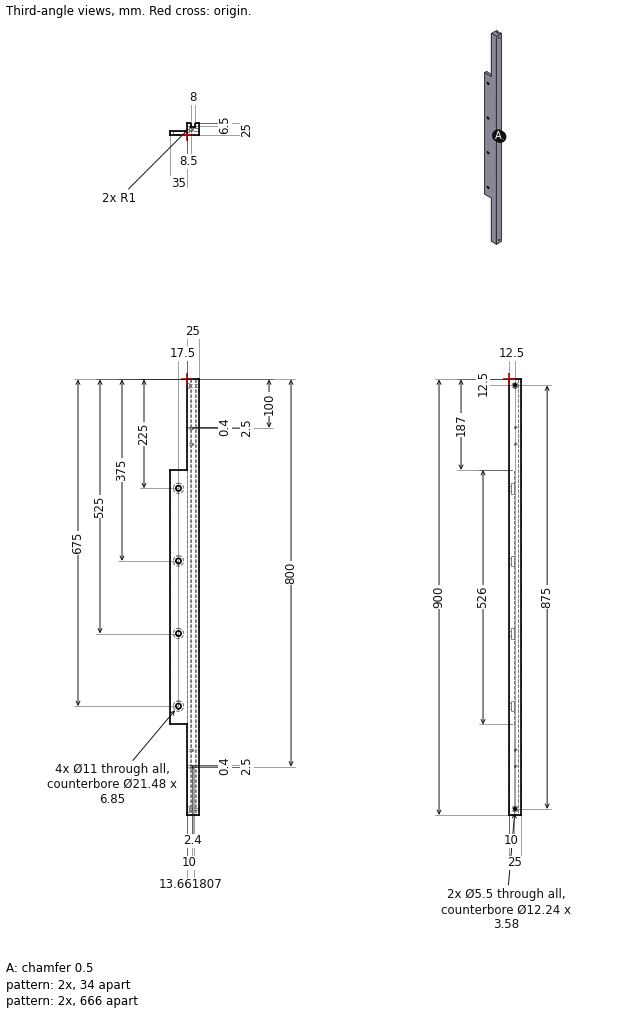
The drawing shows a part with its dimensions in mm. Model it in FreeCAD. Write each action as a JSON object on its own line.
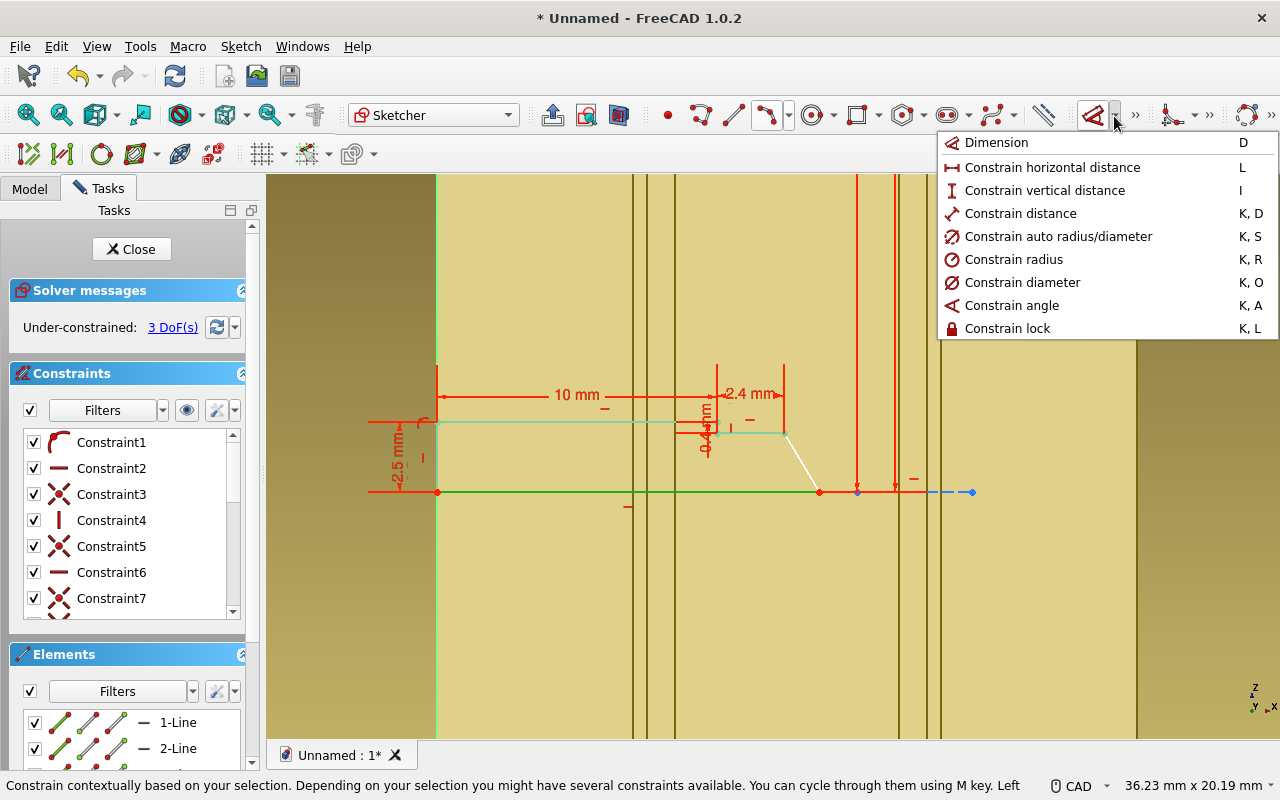
{"action": "left_click", "coordinate": [1108, 168]}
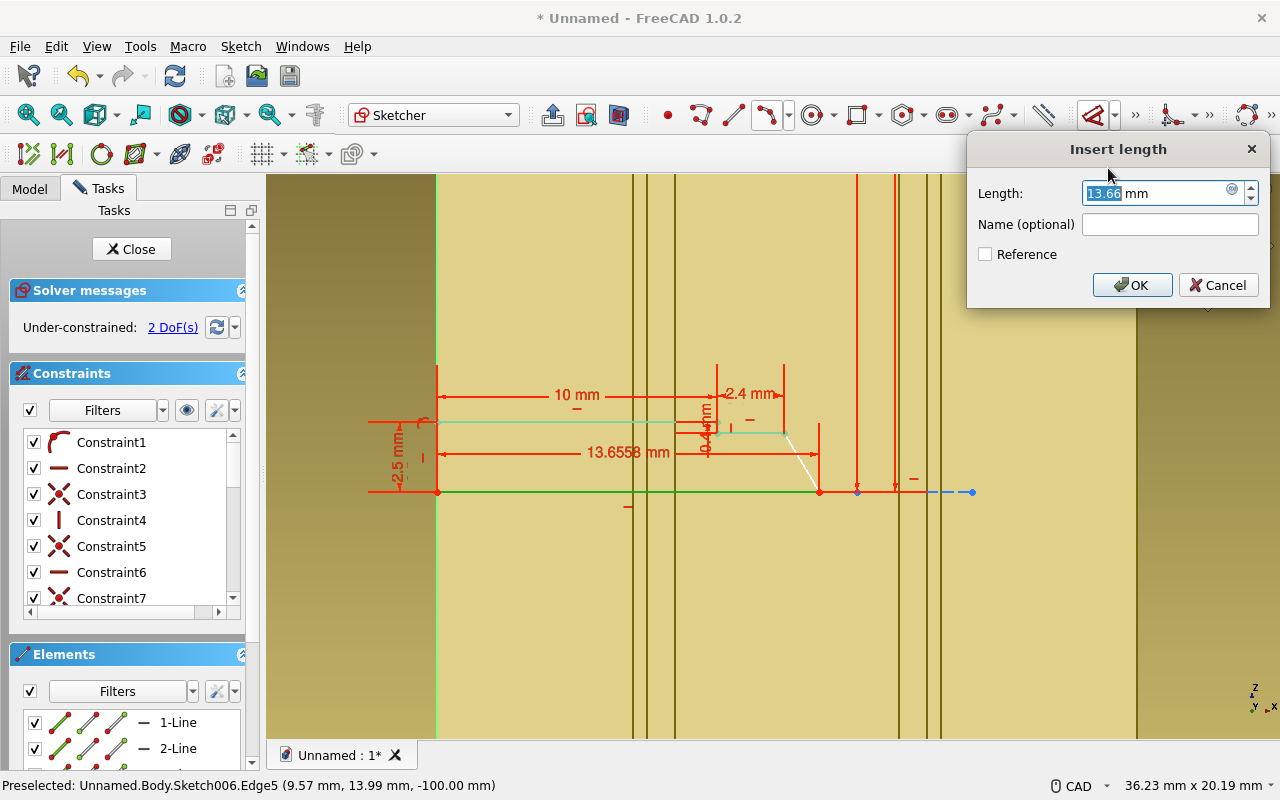
{"action": "type", "text": "13.661807"}
{"action": "key", "text": "Return"}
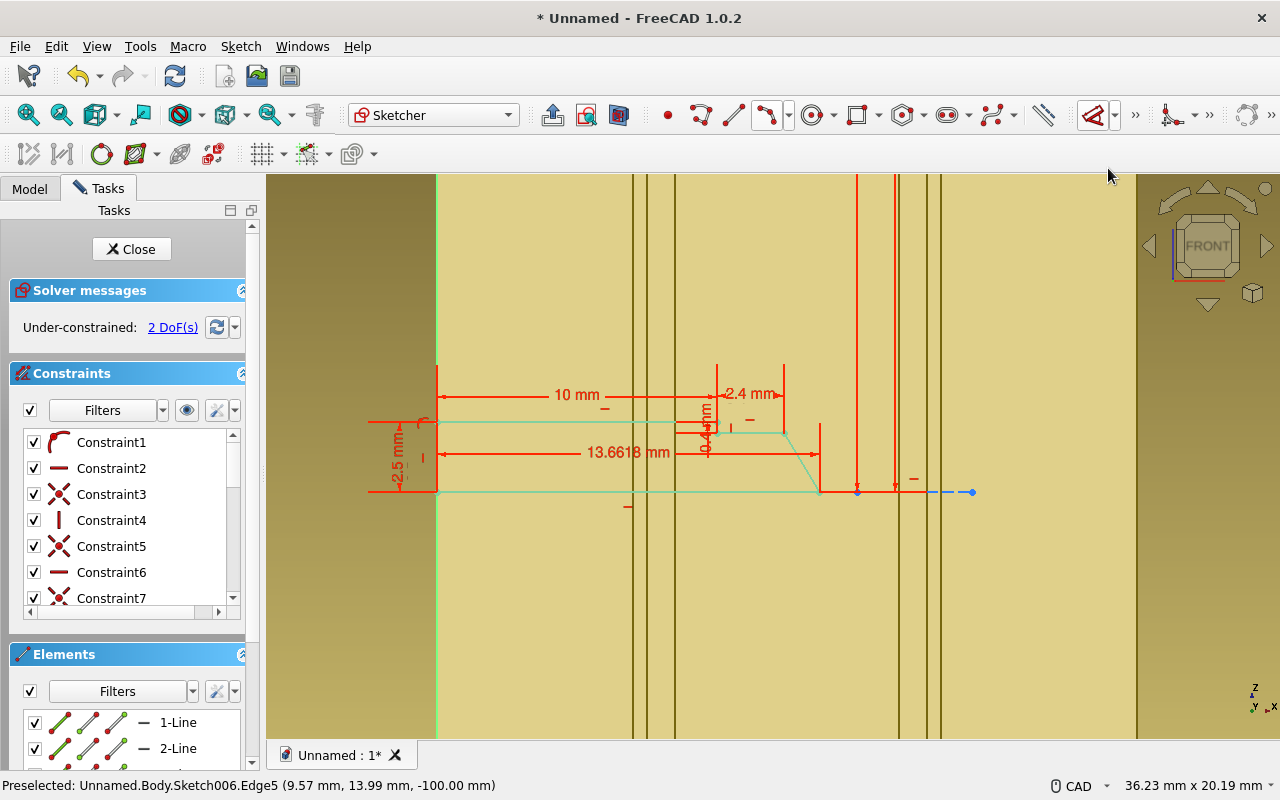
{"action": "left_click", "coordinate": [132, 249]}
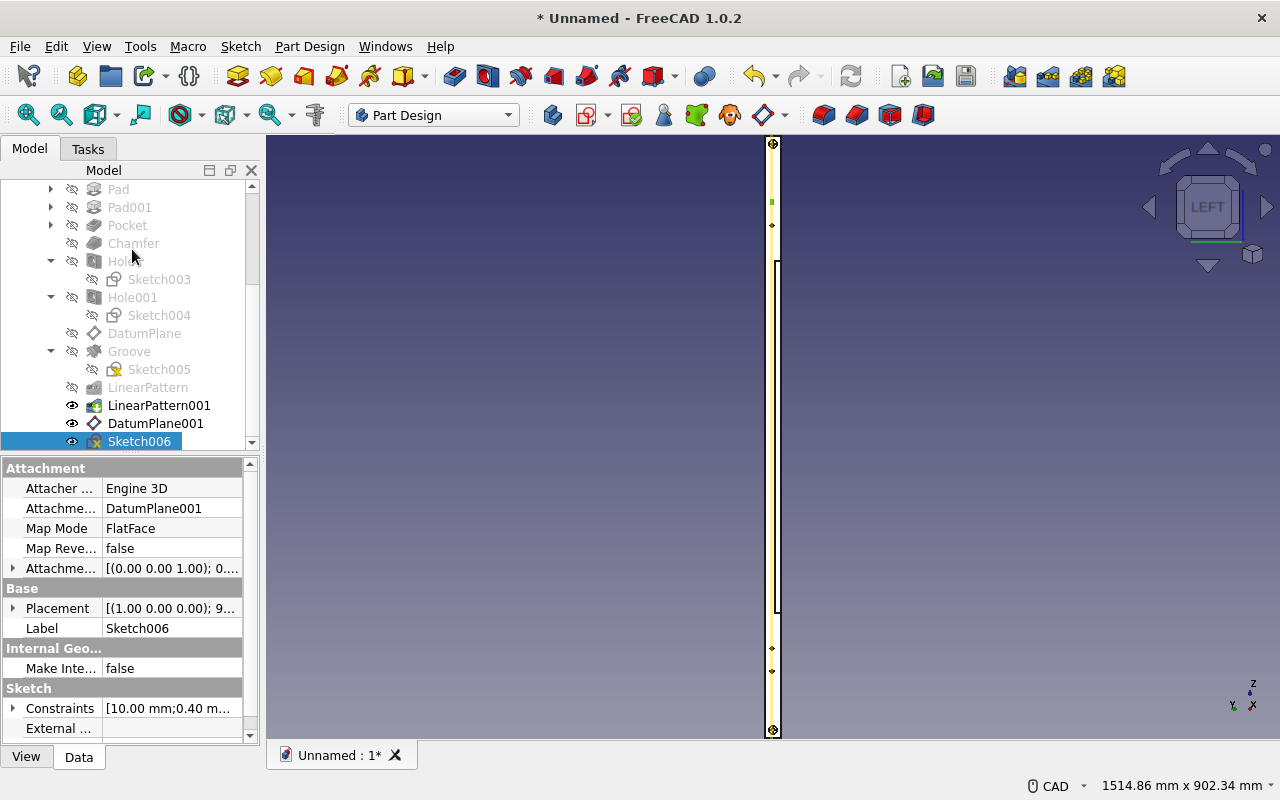
{"action": "left_click", "coordinate": [521, 76]}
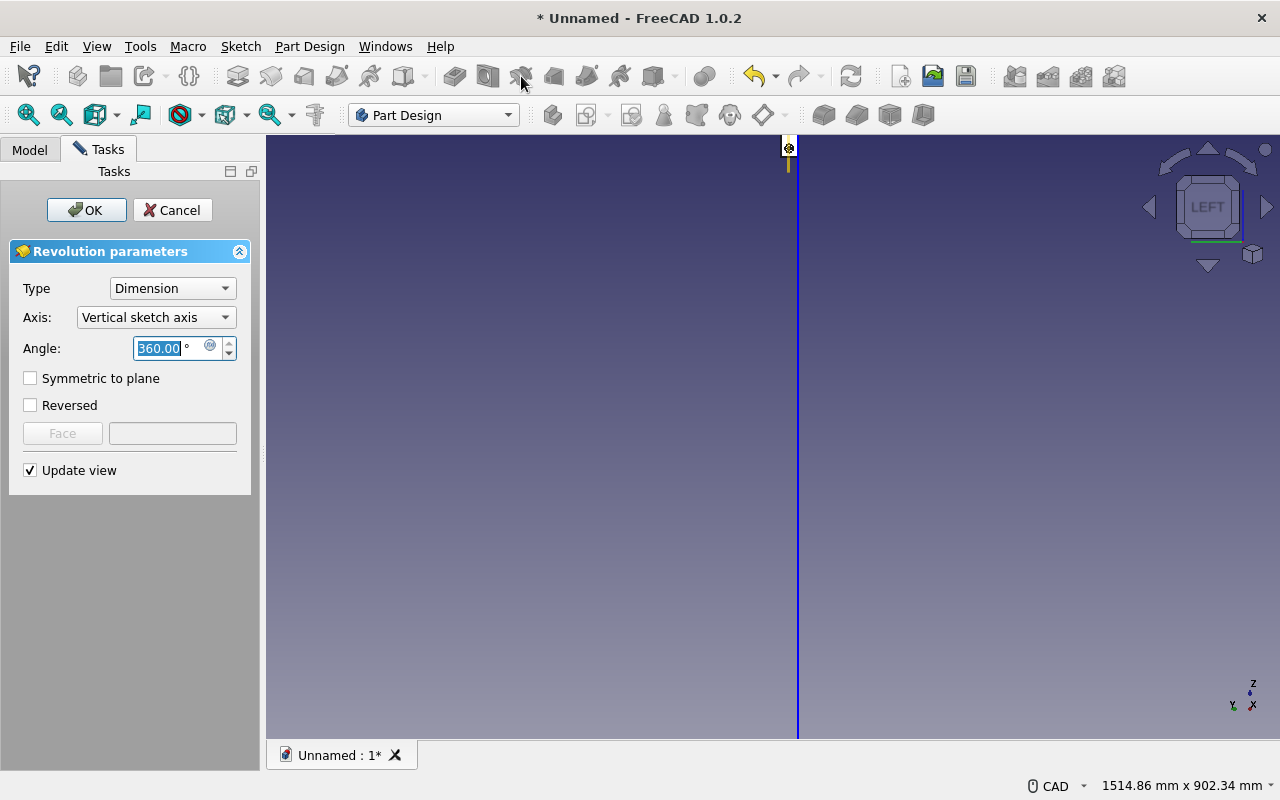
{"action": "left_click", "coordinate": [157, 318]}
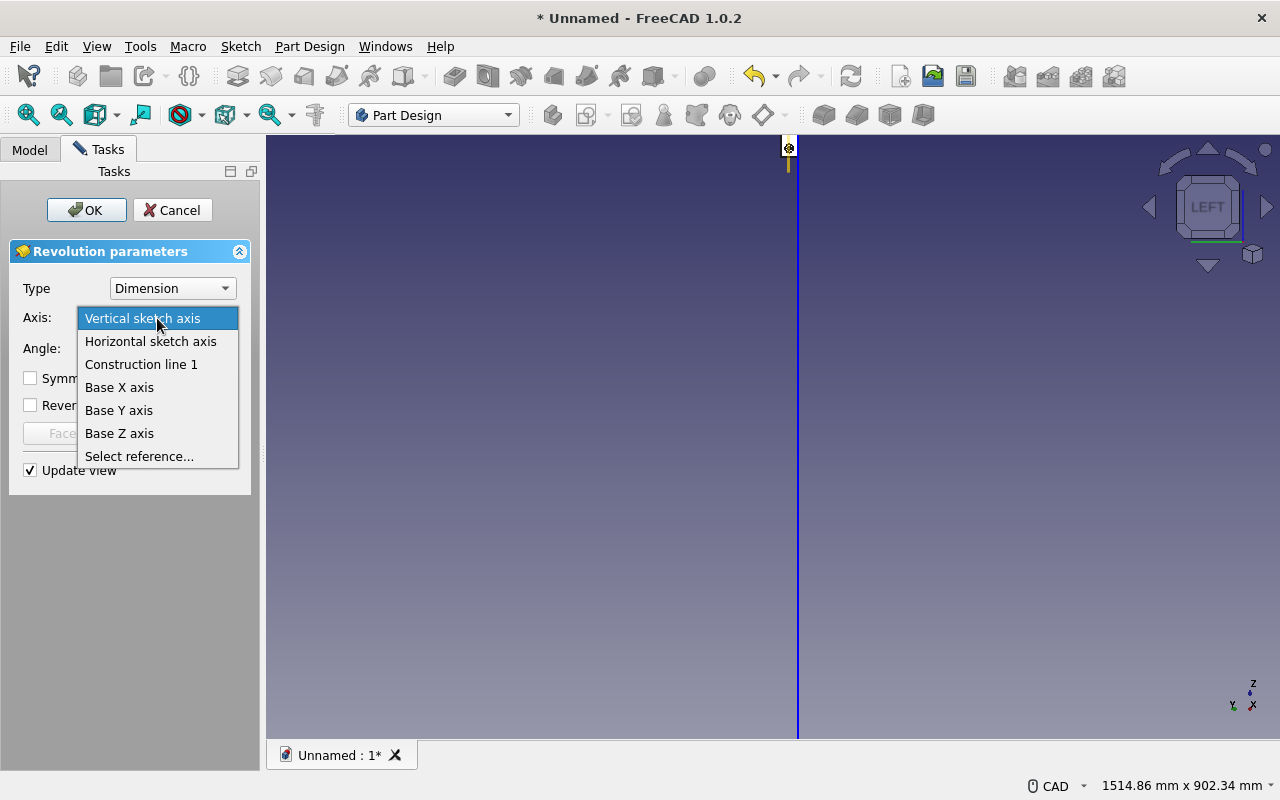
{"action": "left_click", "coordinate": [156, 364]}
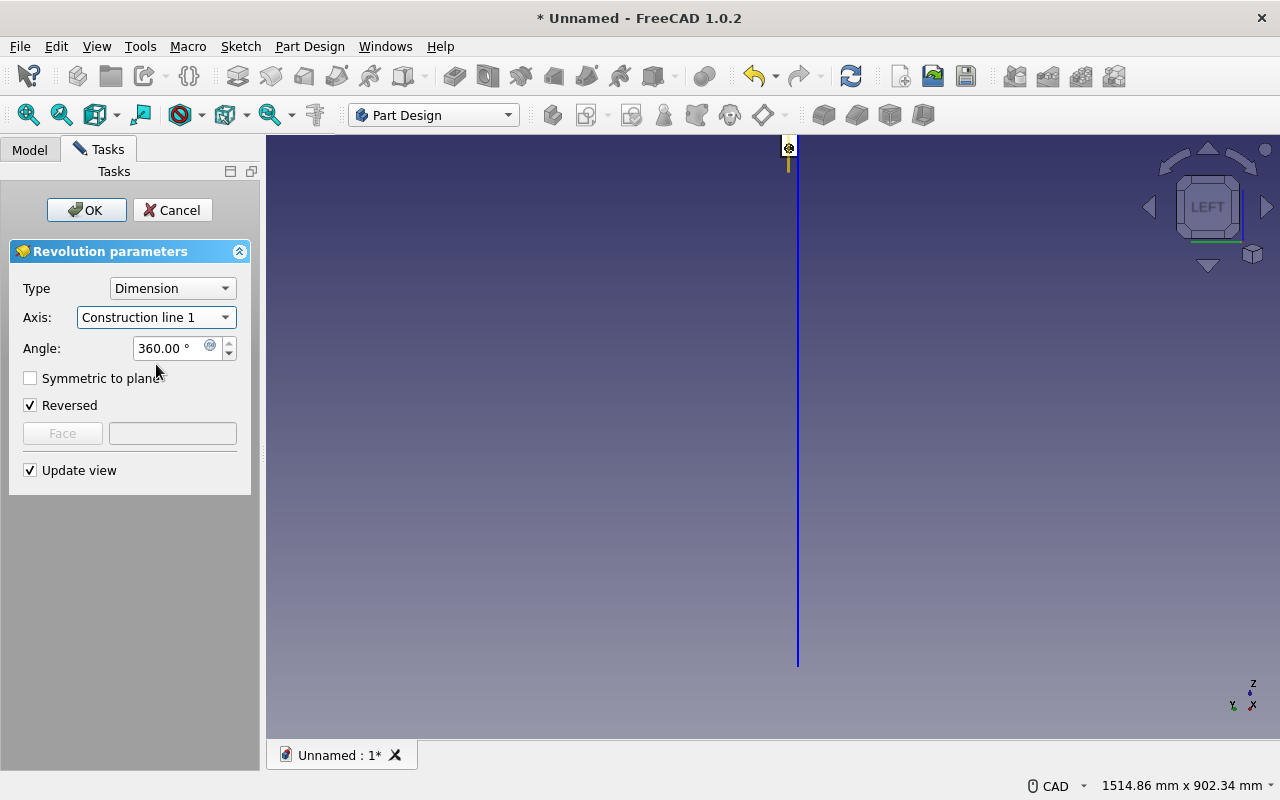
{"action": "left_click", "coordinate": [87, 210]}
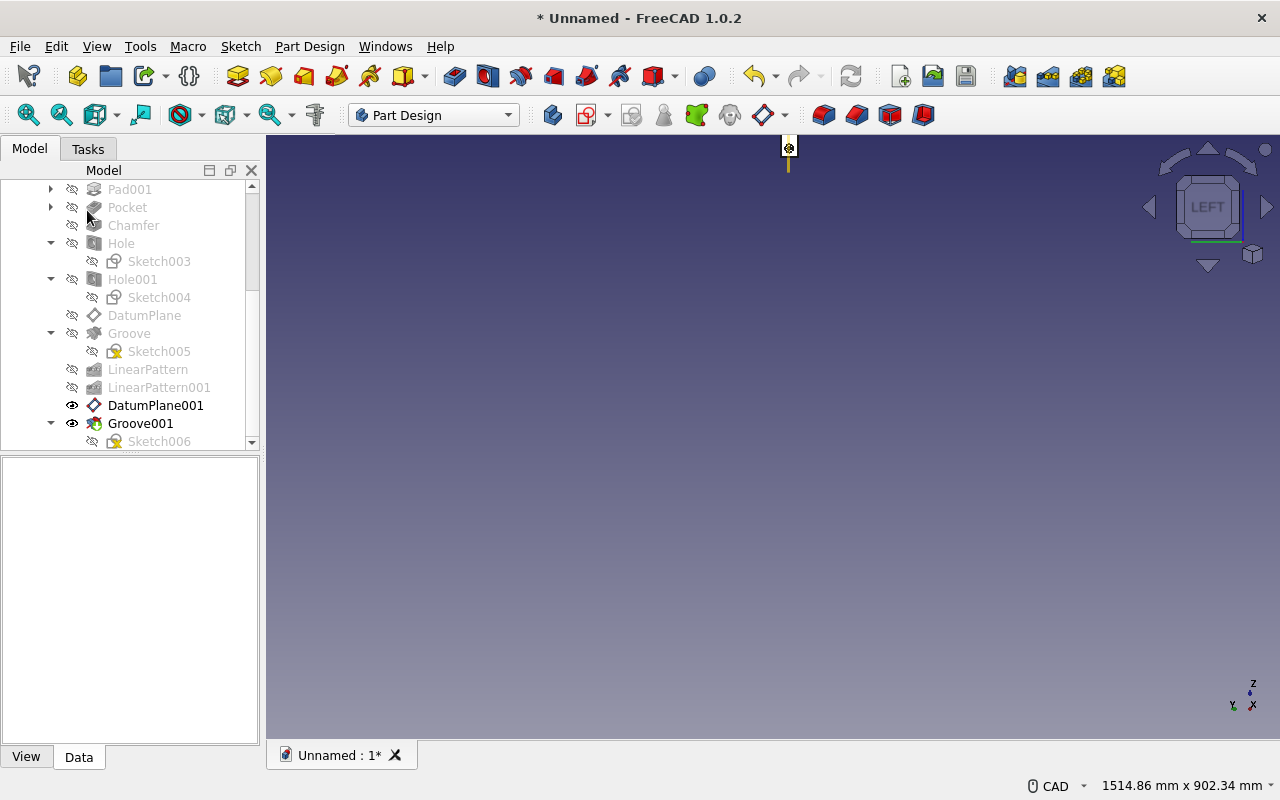
{"action": "left_click", "coordinate": [117, 405]}
{"action": "key", "text": "space"}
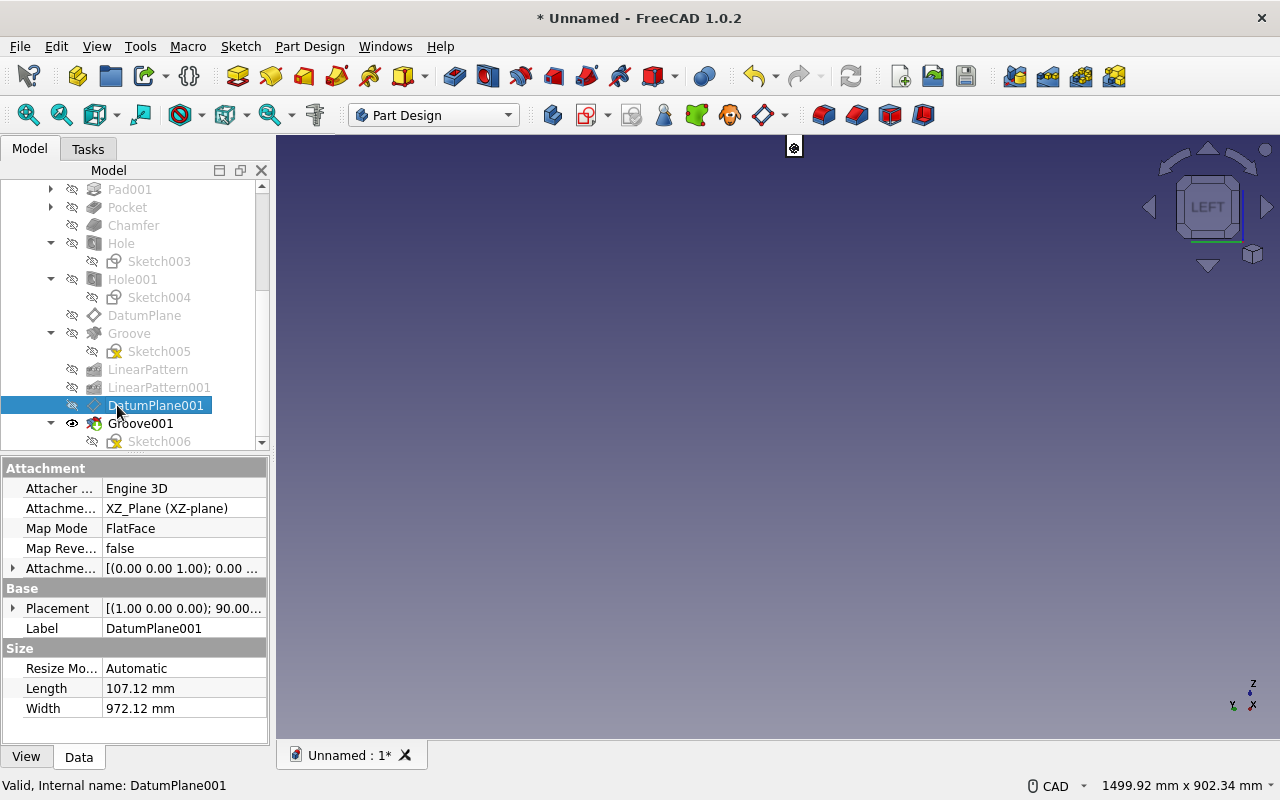
{"action": "key", "text": "0"}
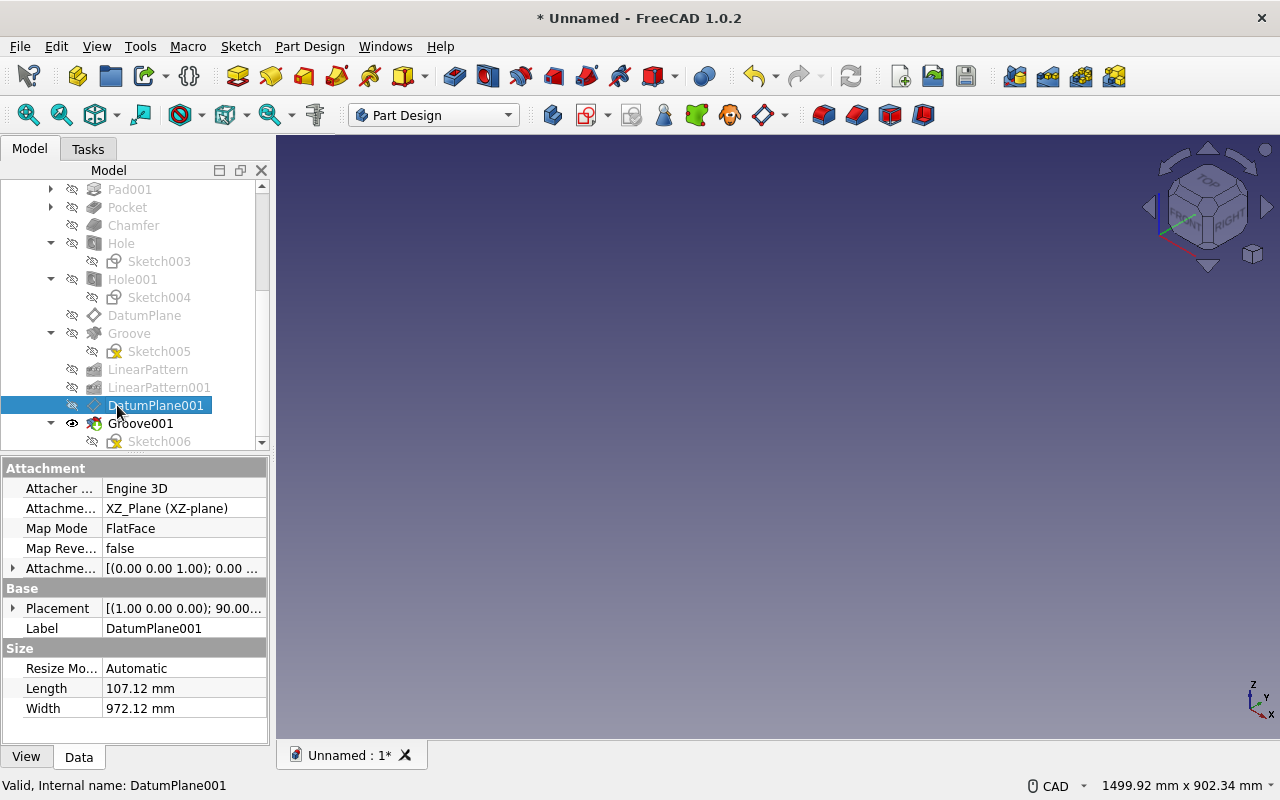
{"action": "left_click", "coordinate": [29, 116]}